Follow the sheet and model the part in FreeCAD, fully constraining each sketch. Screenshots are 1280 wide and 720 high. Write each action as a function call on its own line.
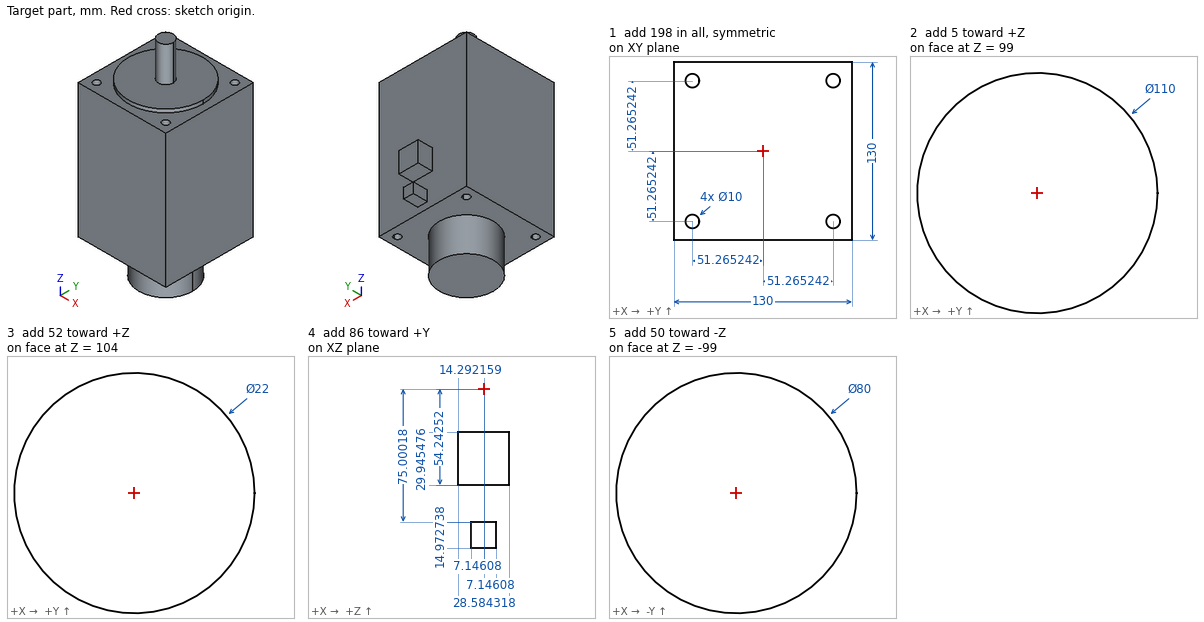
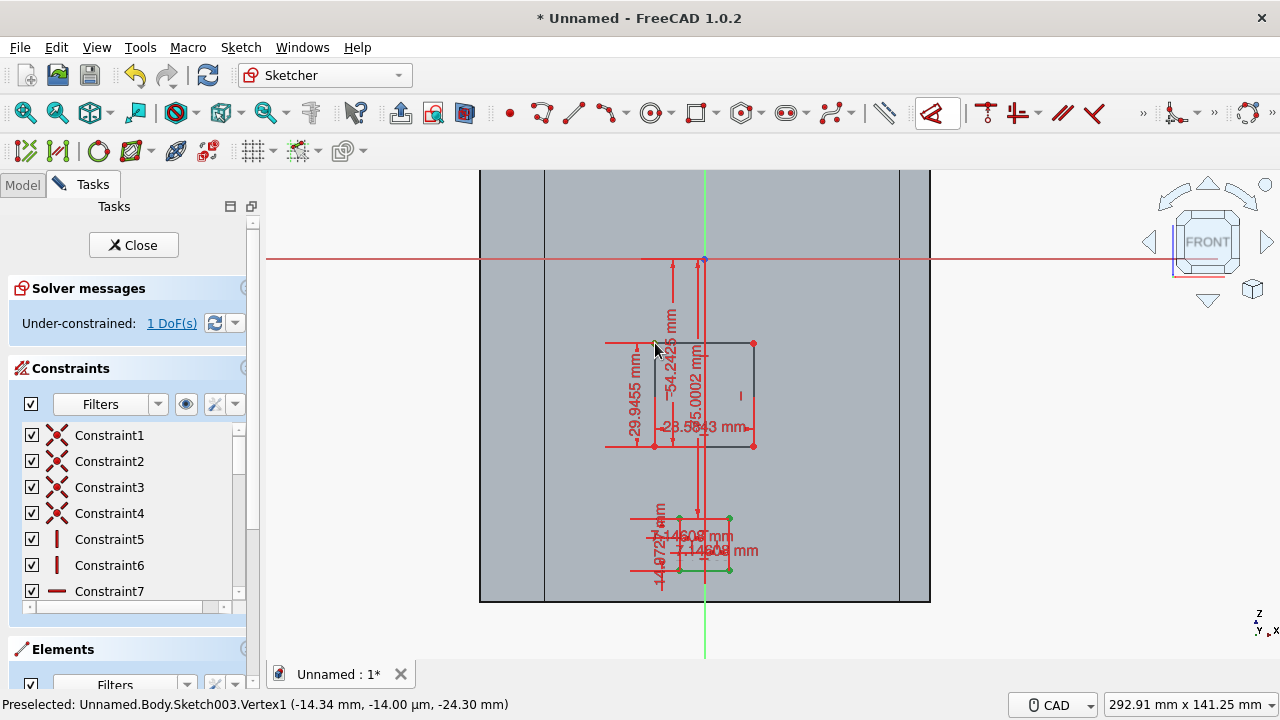
key(l)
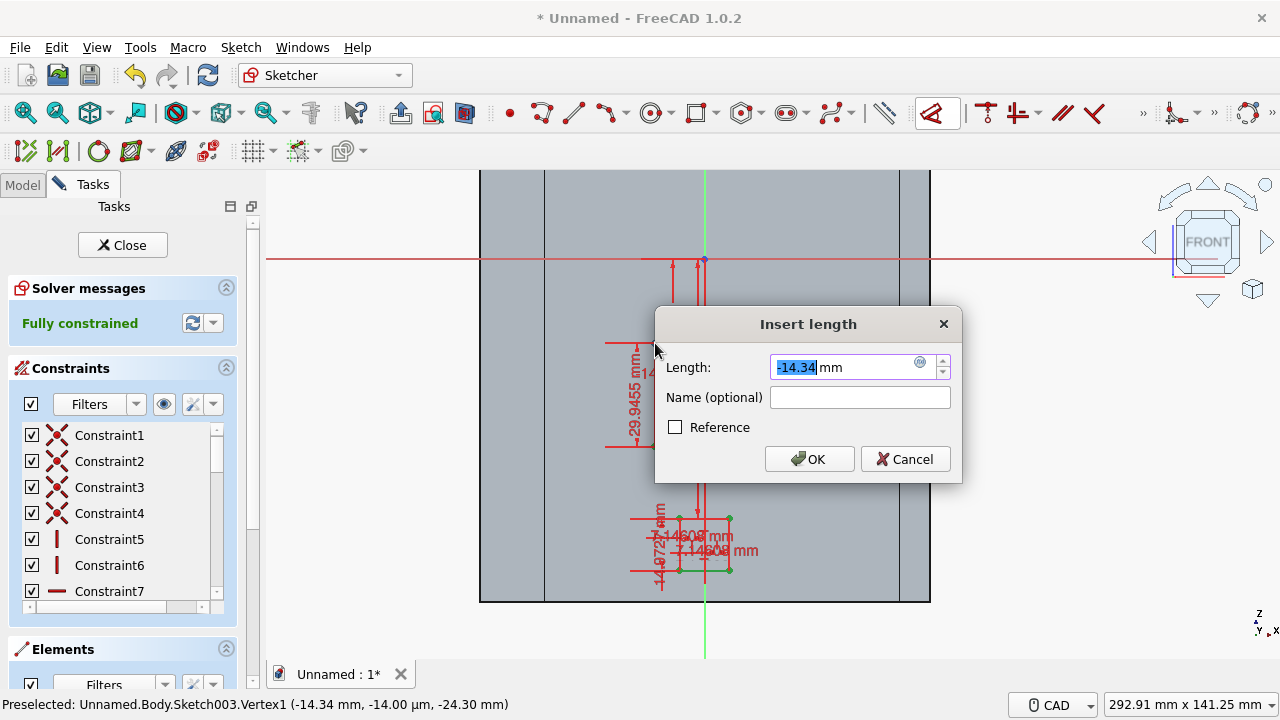
text(-14.292159)
key(Return)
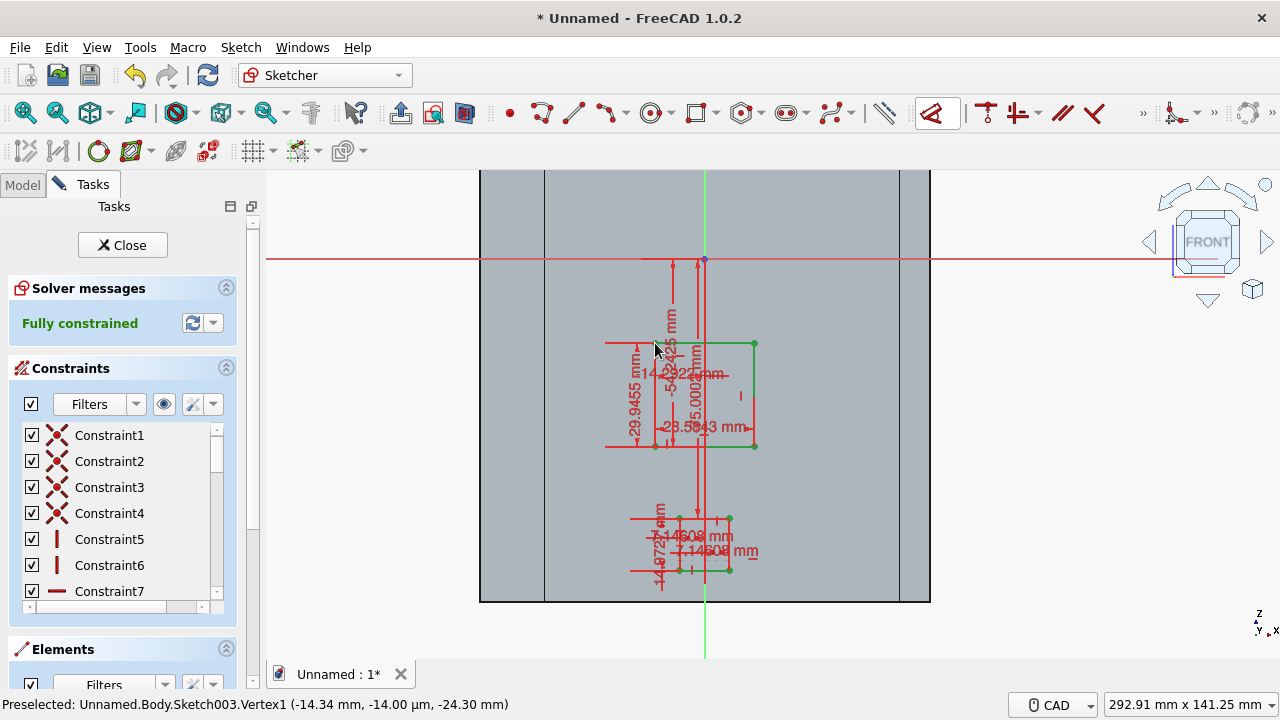
click(123, 245)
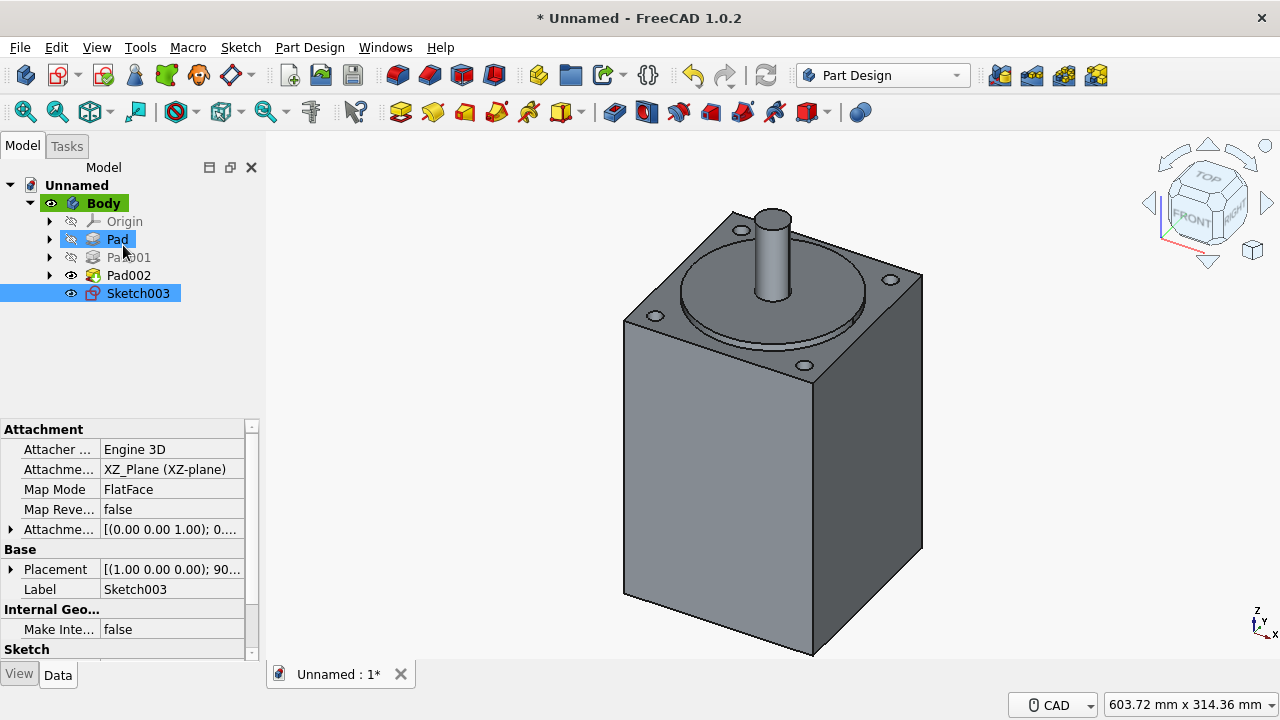
click(402, 112)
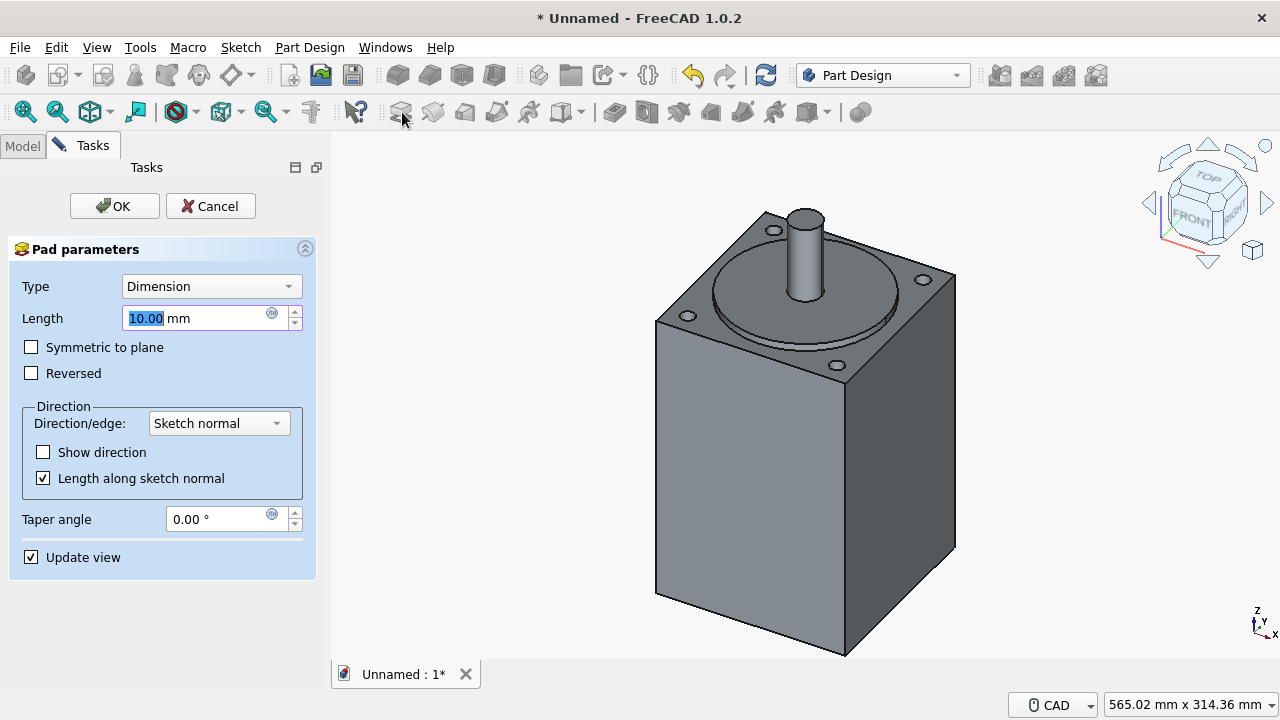
text(86)
key(Tab)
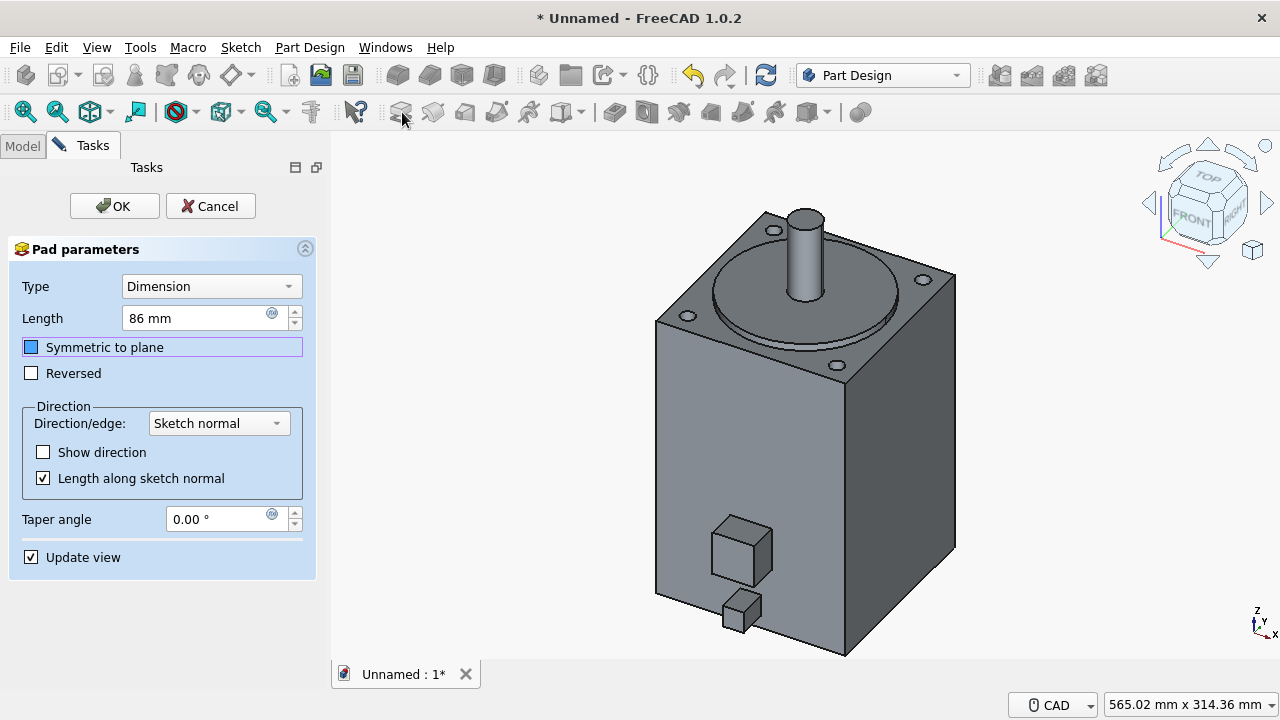
click(30, 373)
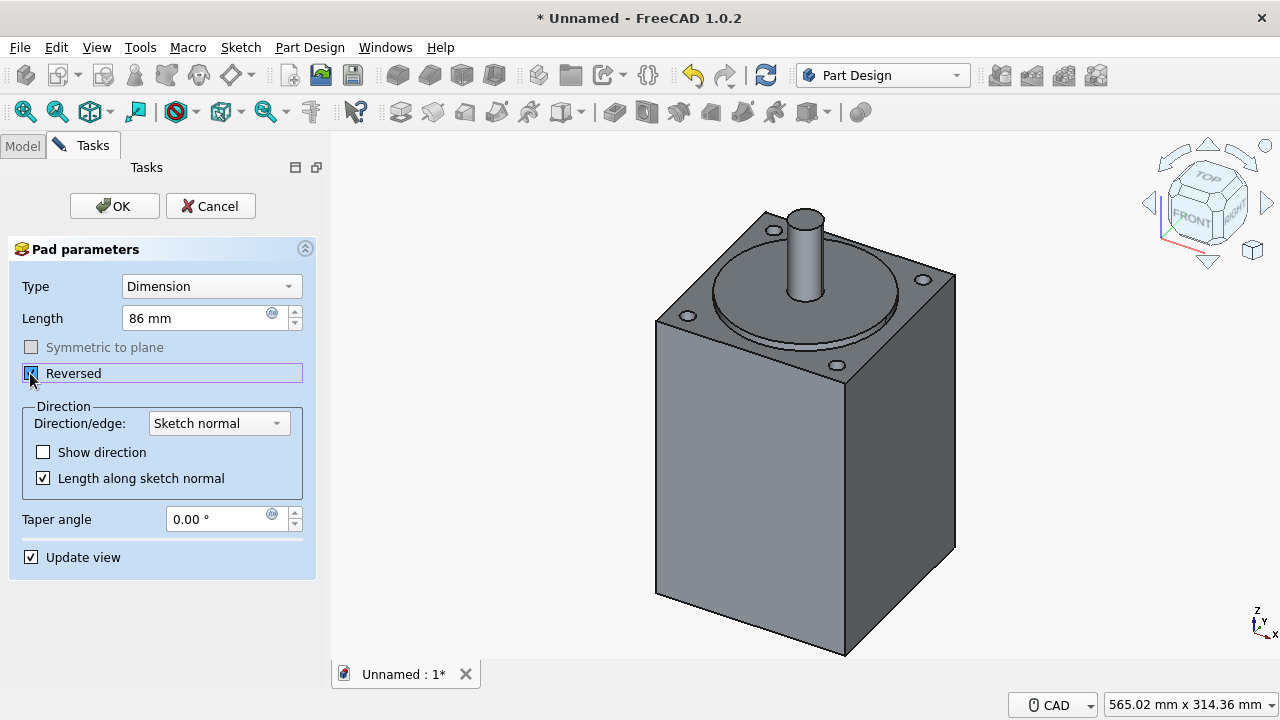
click(115, 206)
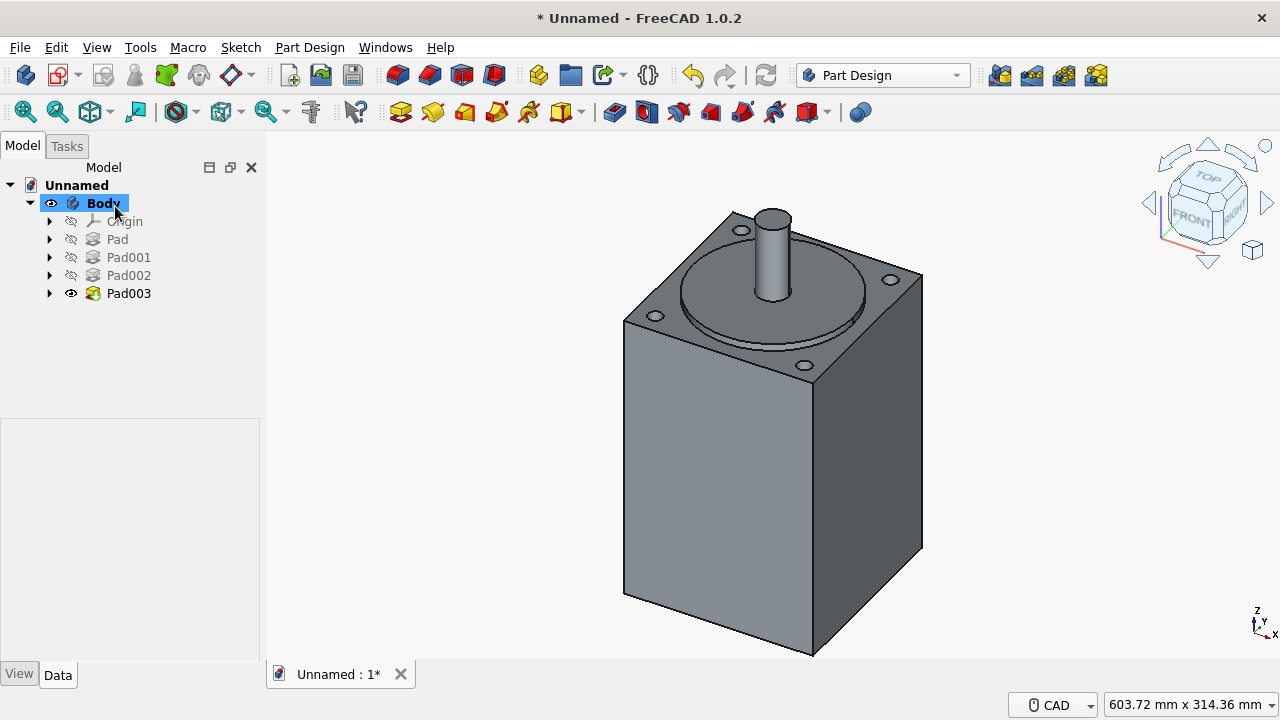
key(v)
key(f)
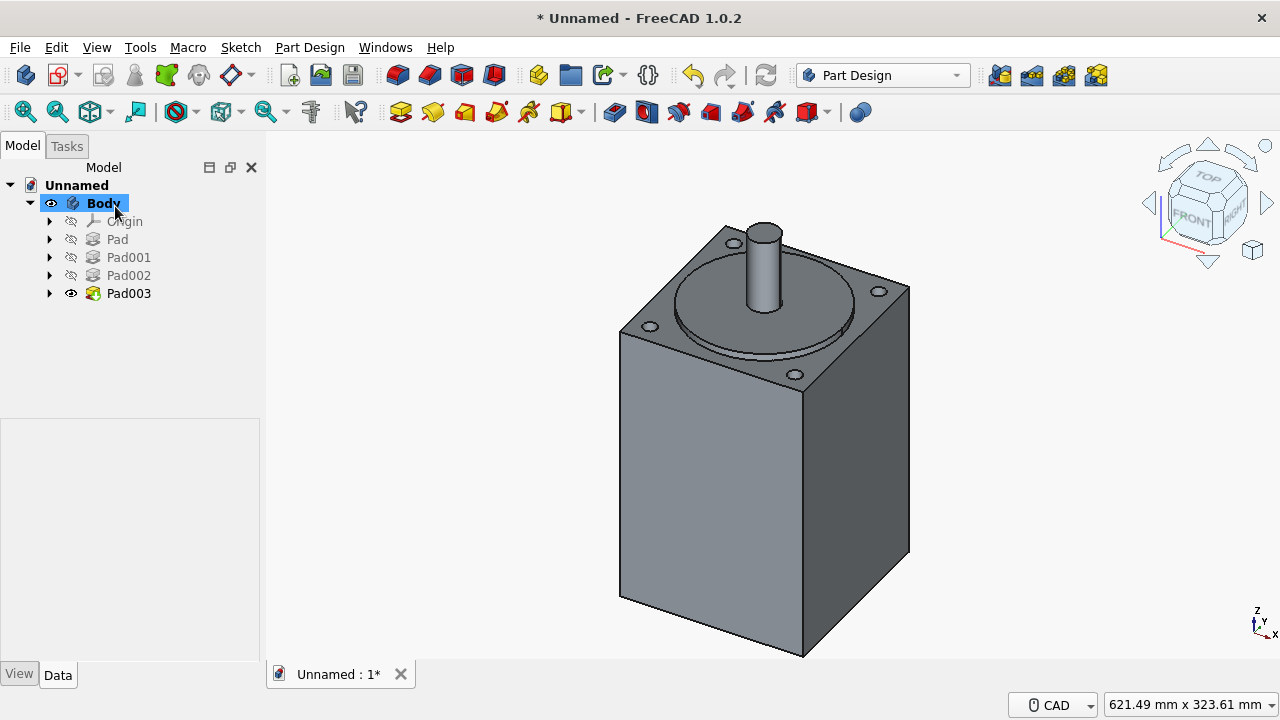
key(5)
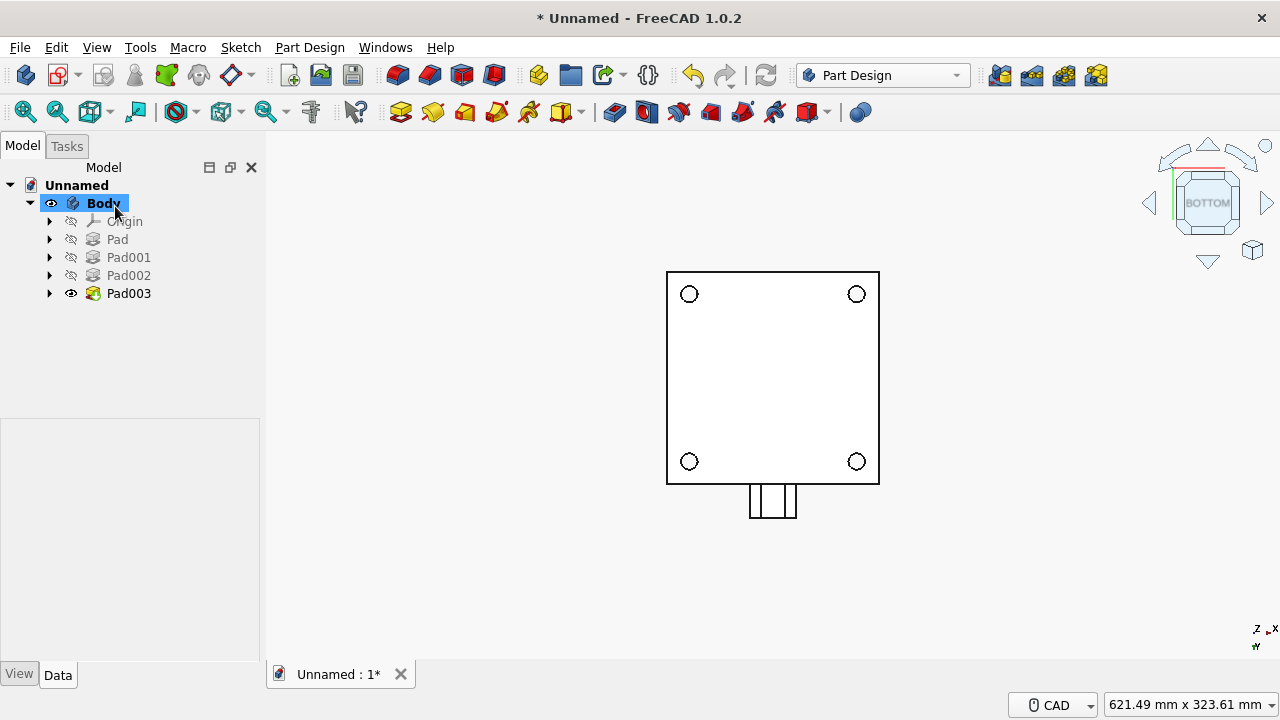
click(773, 377)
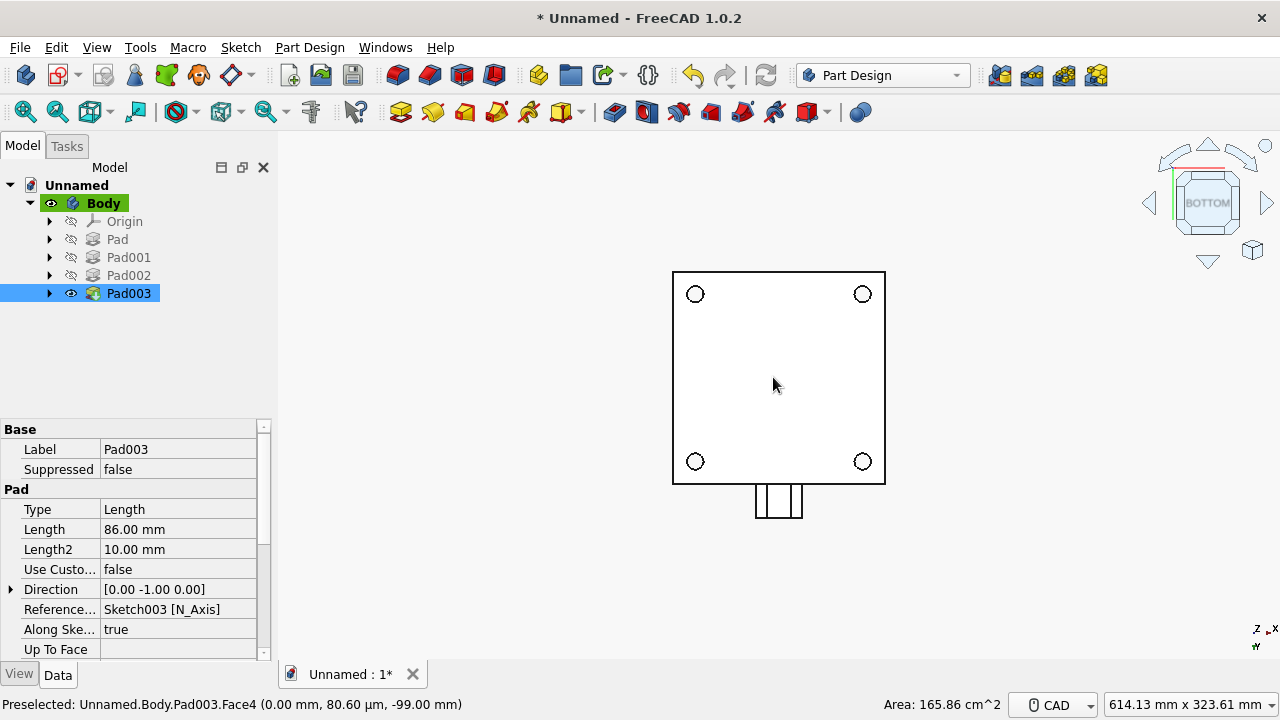
click(58, 76)